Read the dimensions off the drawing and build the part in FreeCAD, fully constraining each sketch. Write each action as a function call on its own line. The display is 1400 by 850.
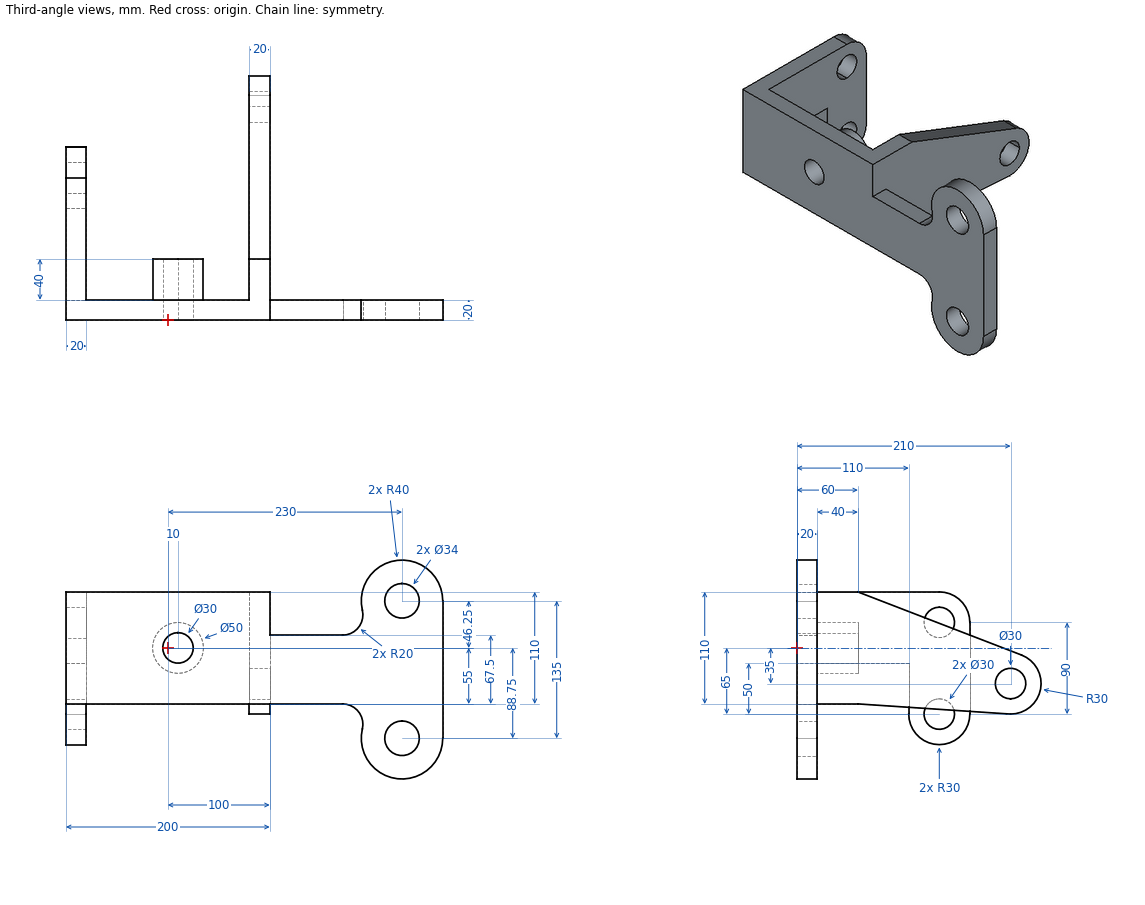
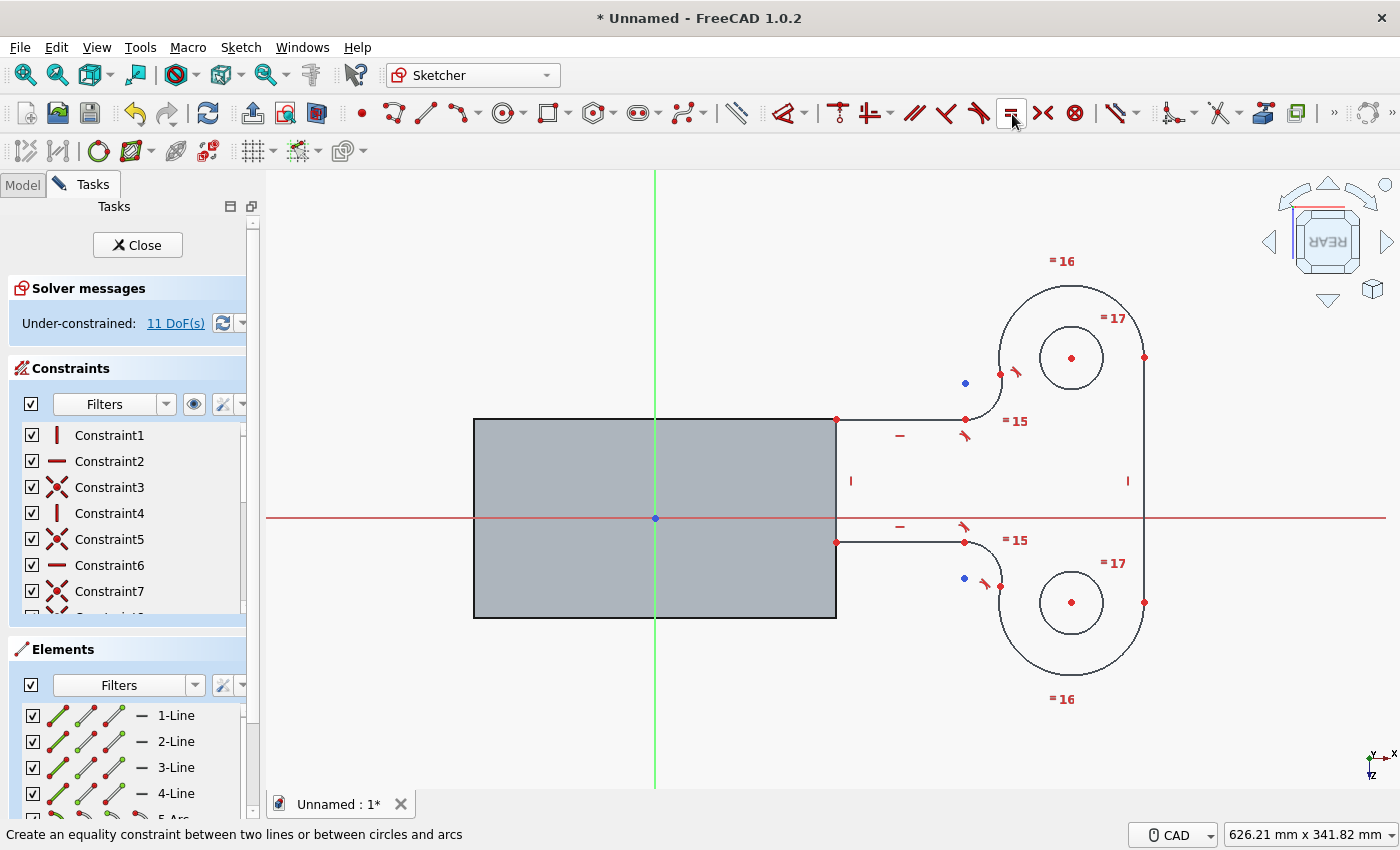
click(1110, 297)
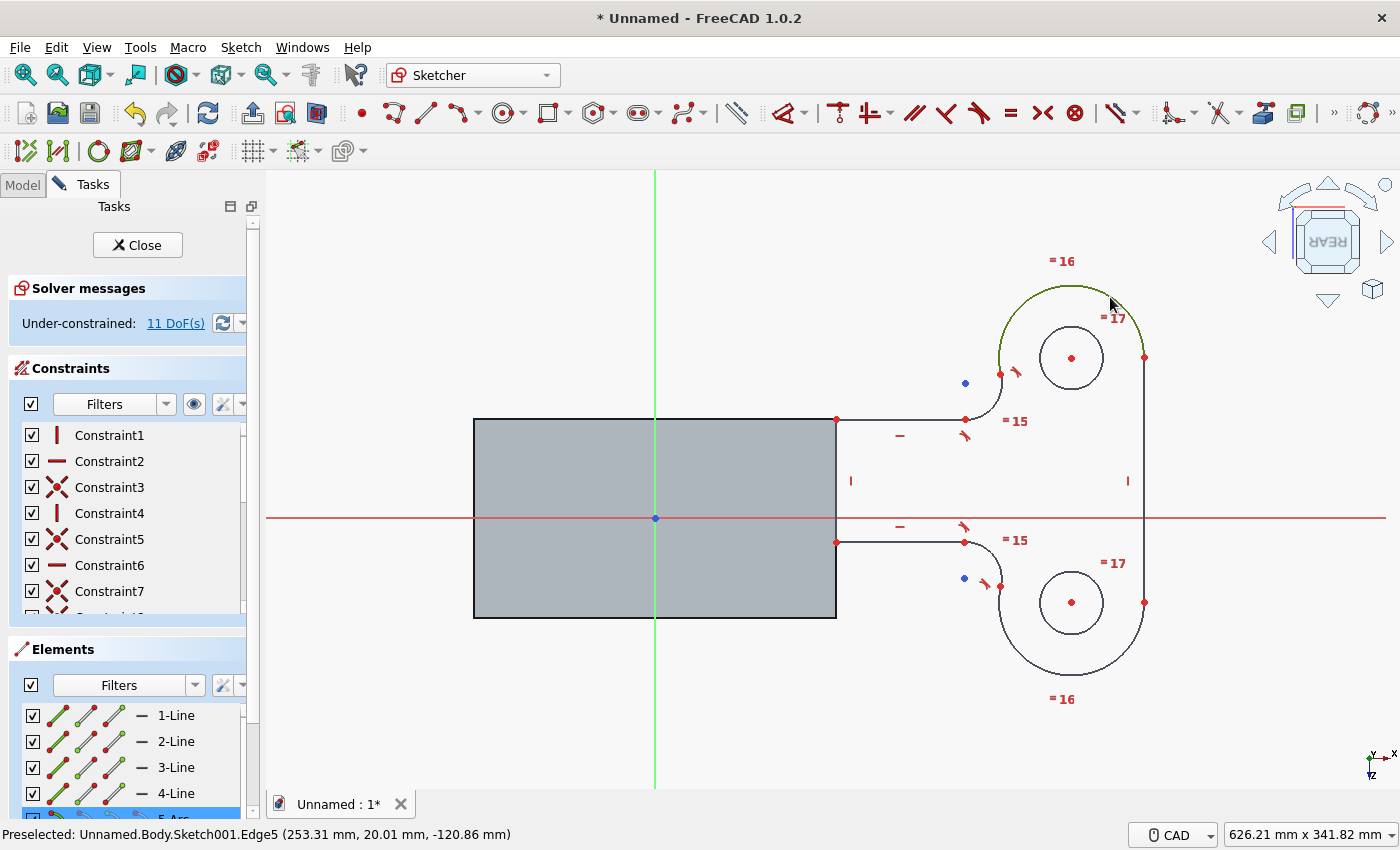
key(k)
key(r)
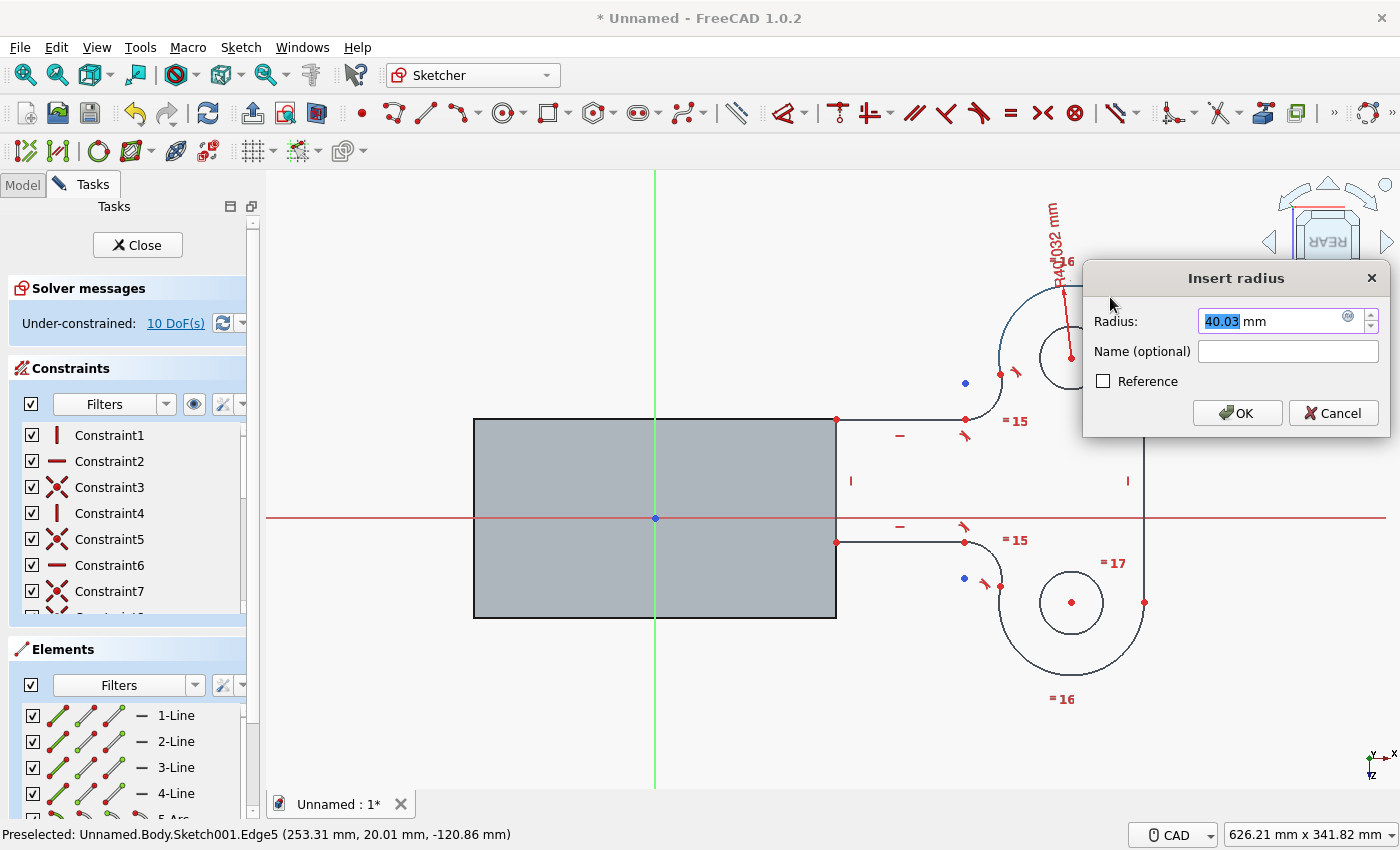
text(40)
key(Return)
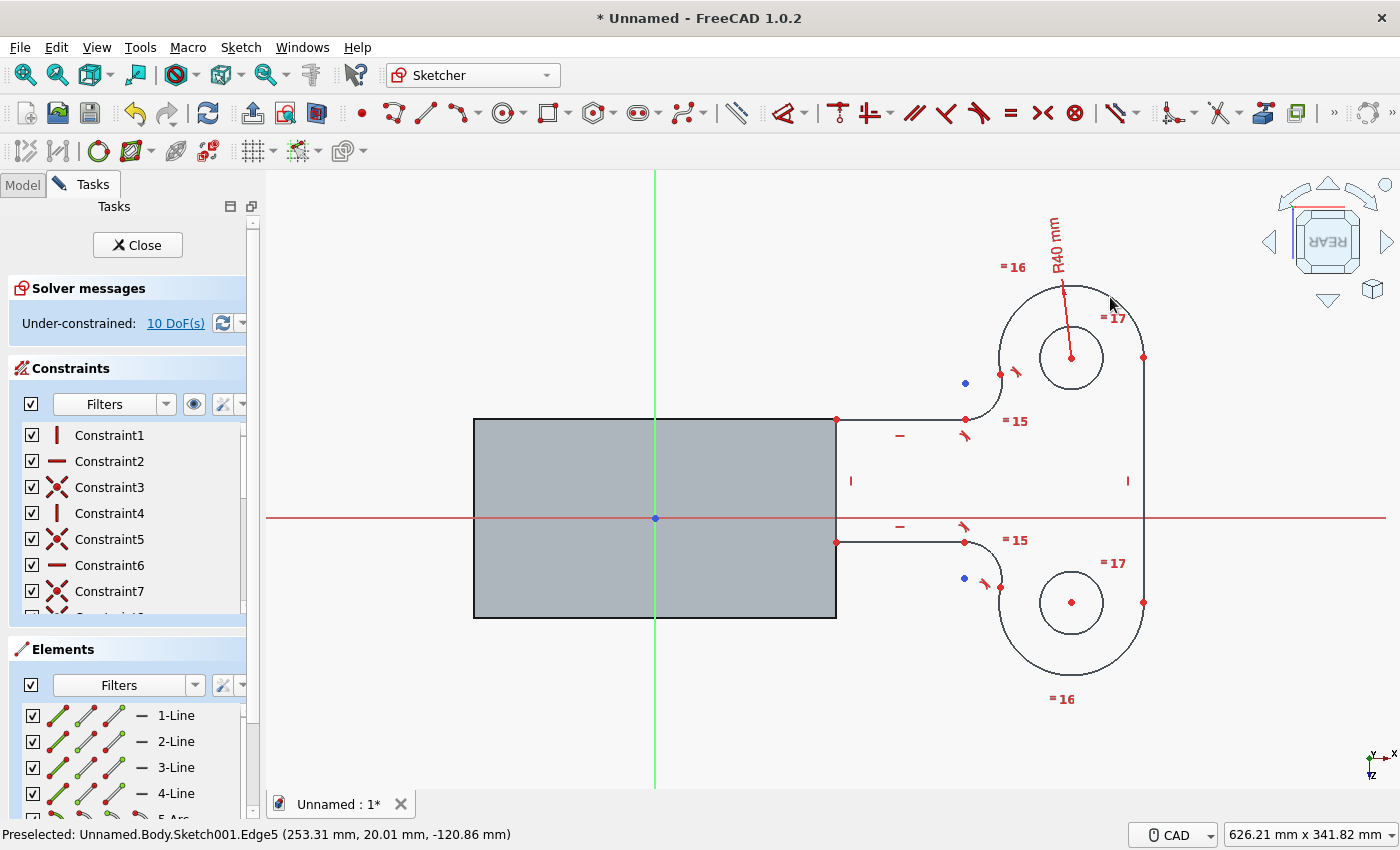
click(984, 415)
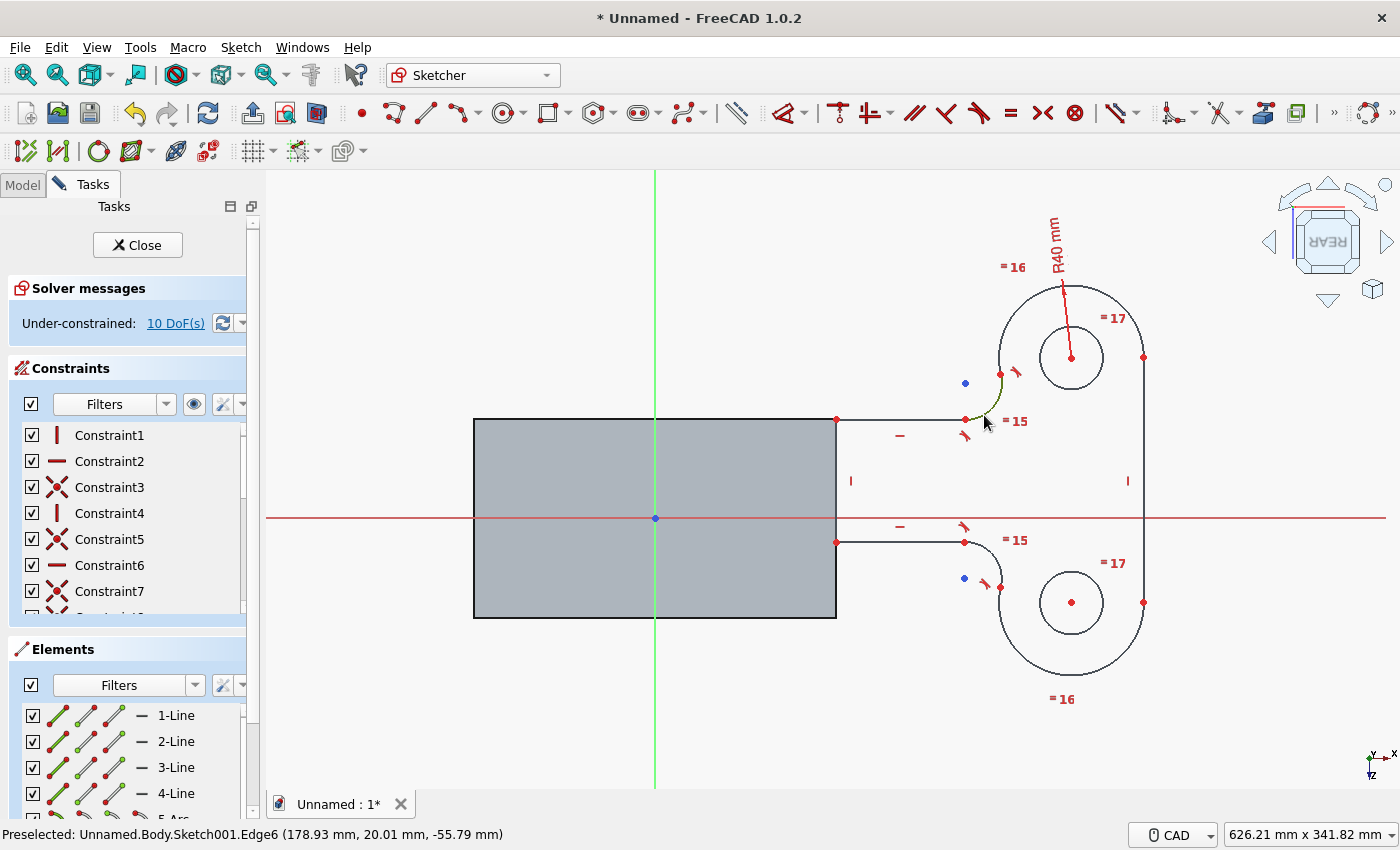
key(k)
key(r)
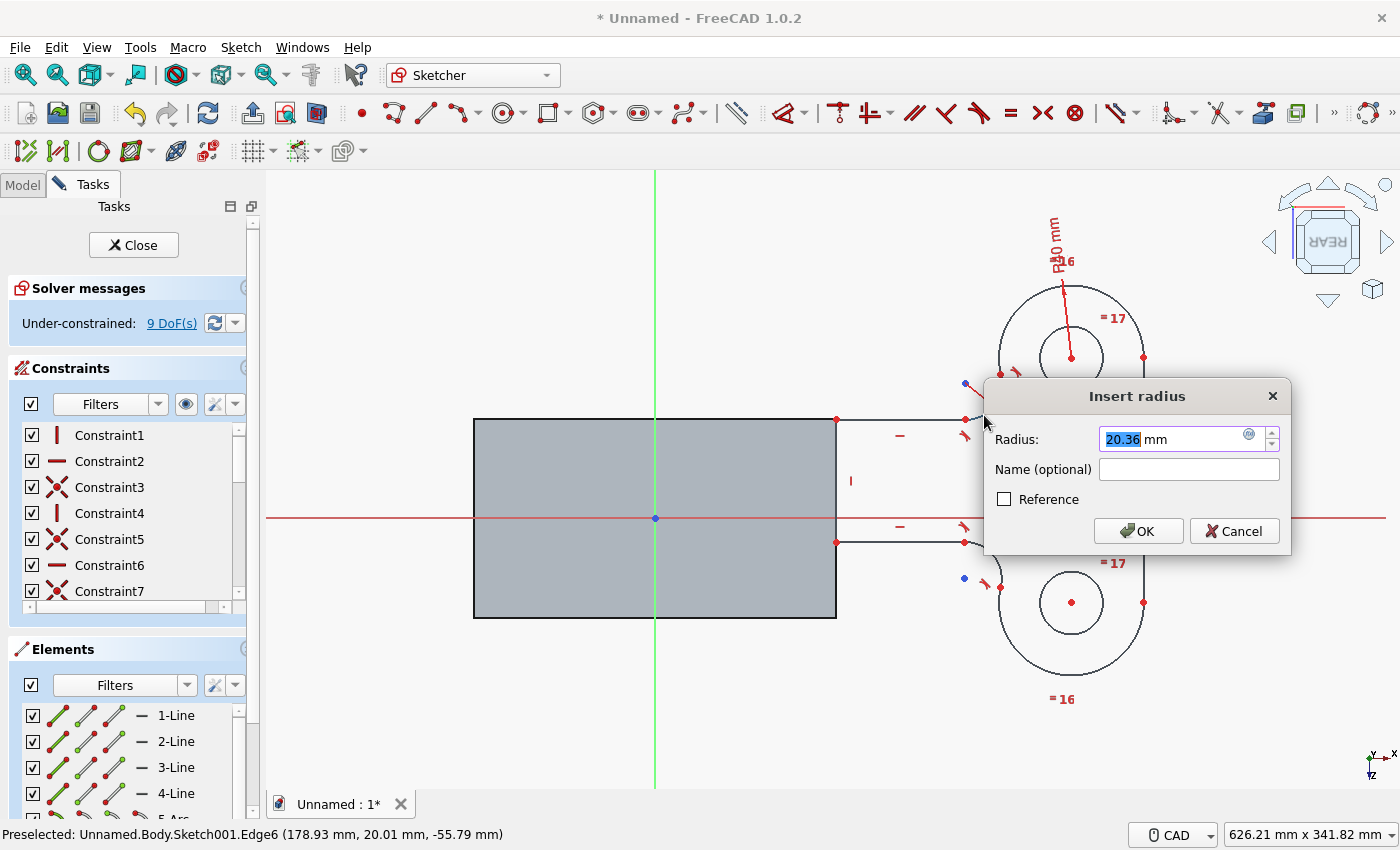
text(20)
key(Return)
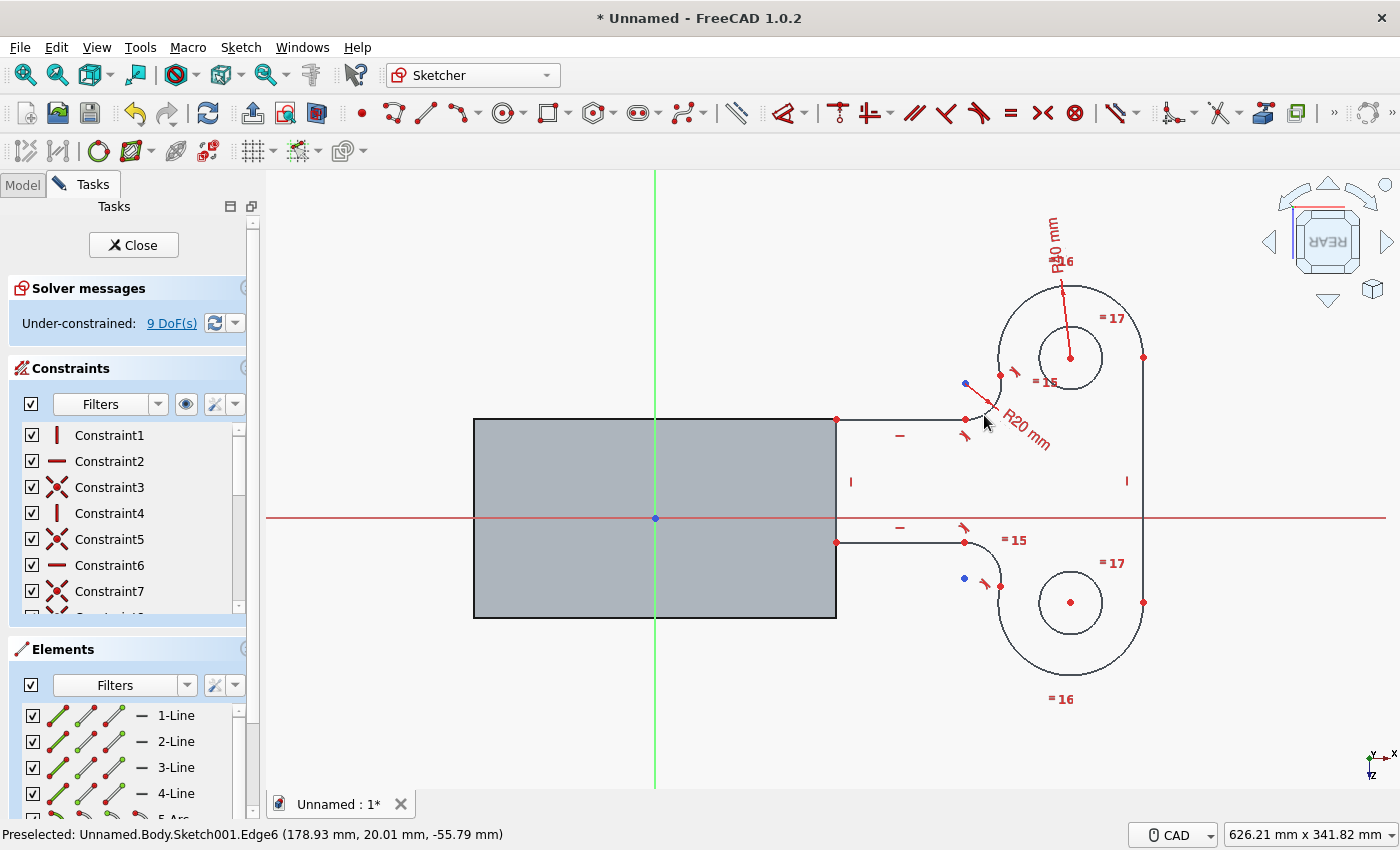
click(1093, 581)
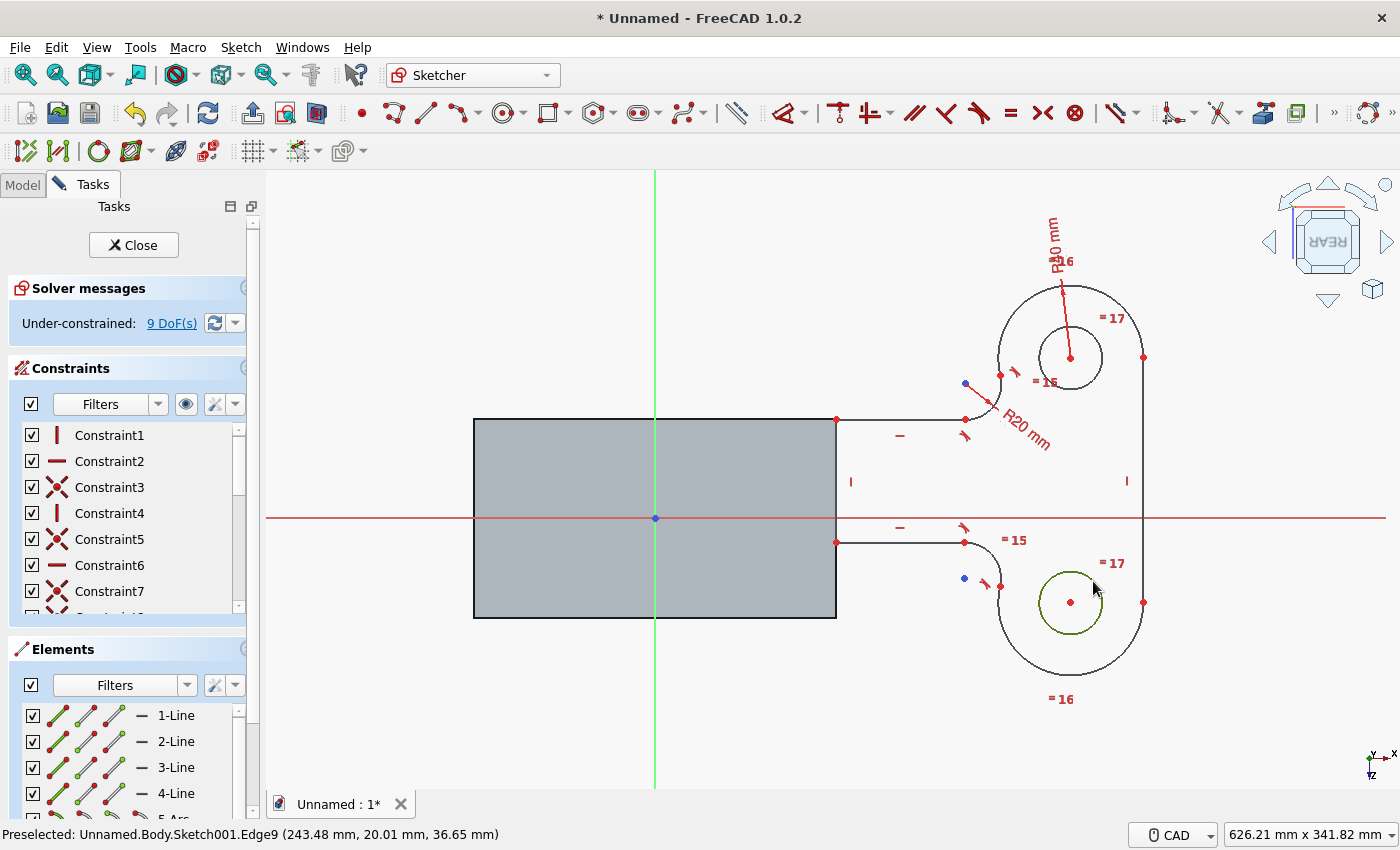
key(k)
key(o)